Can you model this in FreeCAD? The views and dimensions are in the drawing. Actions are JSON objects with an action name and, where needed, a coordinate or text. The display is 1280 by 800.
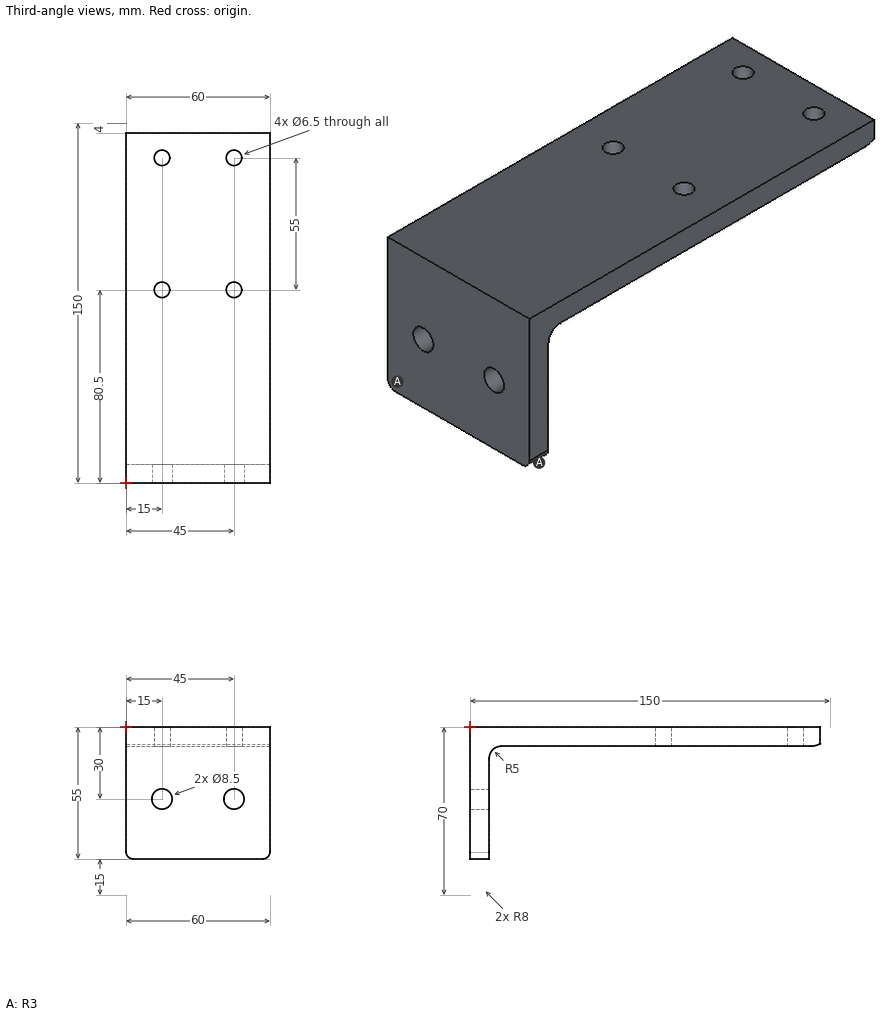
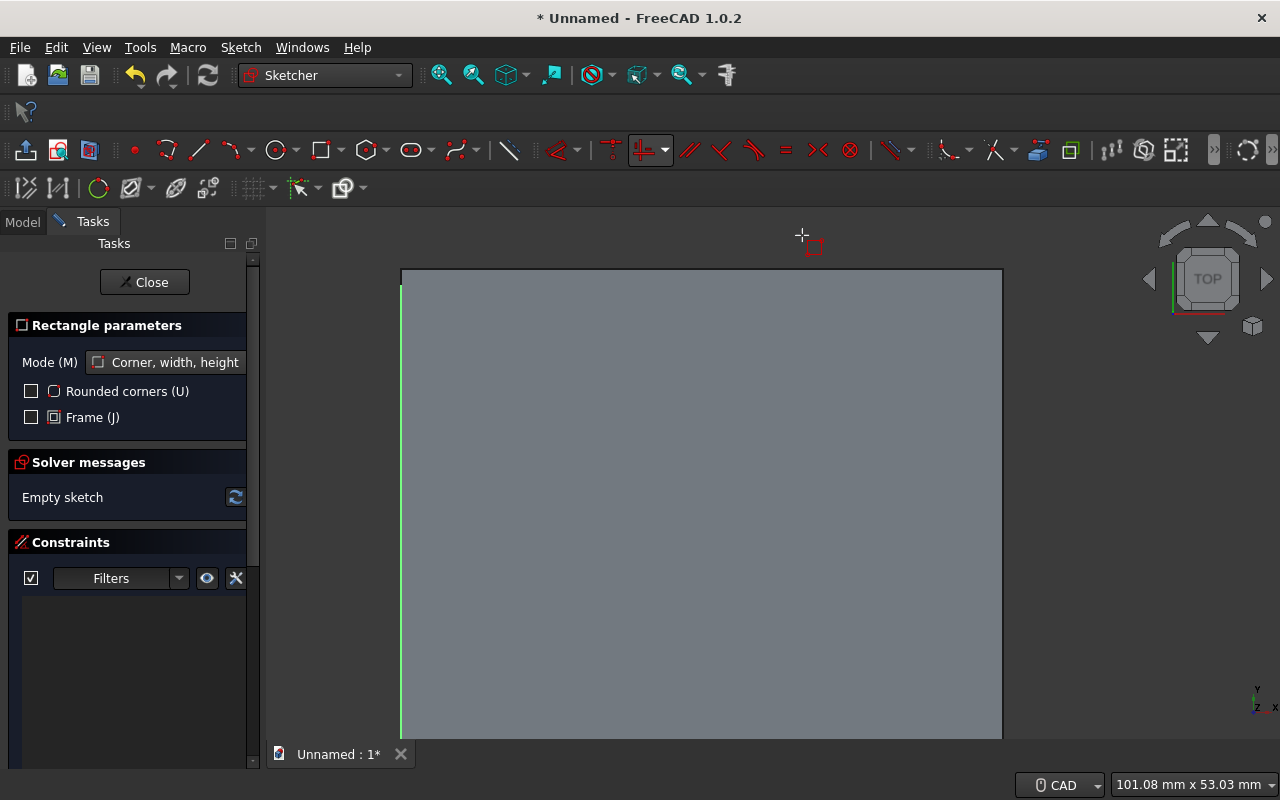
{"action": "left_click", "coordinate": [401, 269]}
{"action": "left_click", "coordinate": [1003, 309]}
{"action": "key", "text": "Escape"}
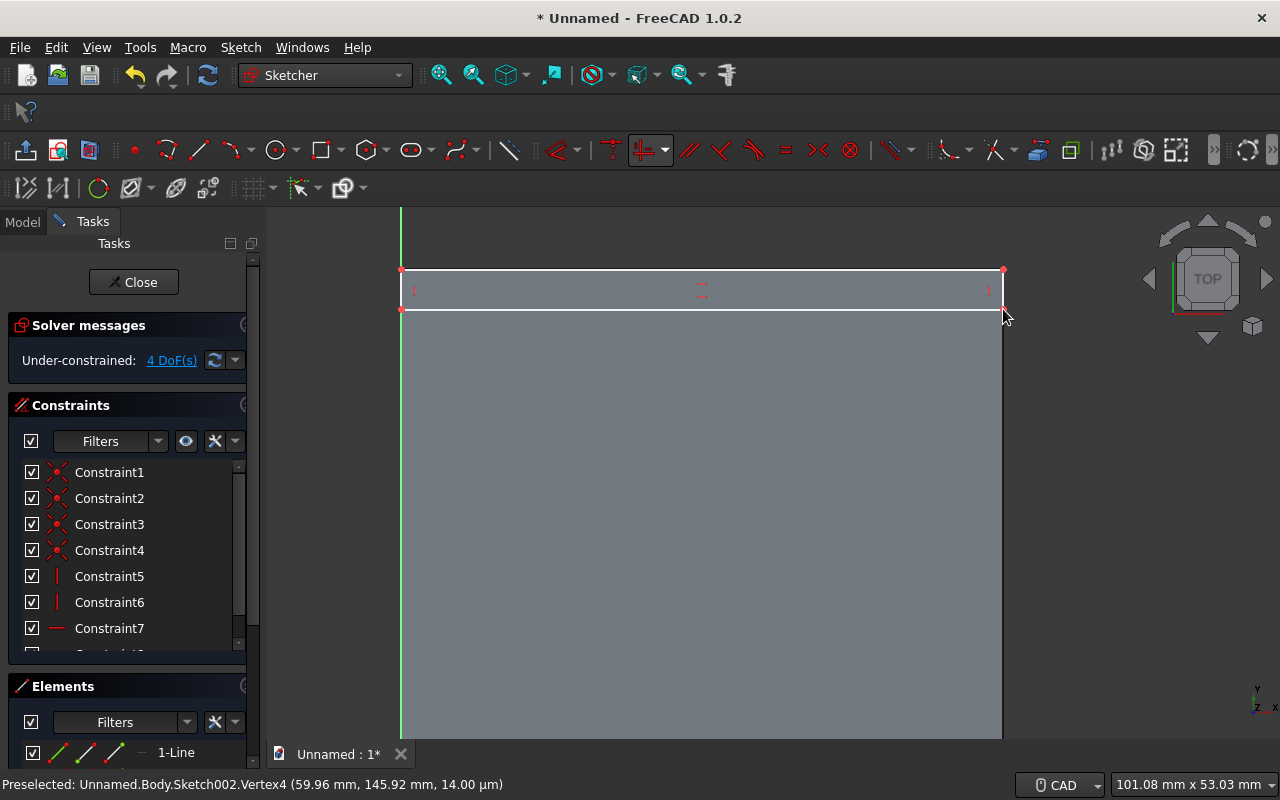
{"action": "left_click", "coordinate": [401, 270]}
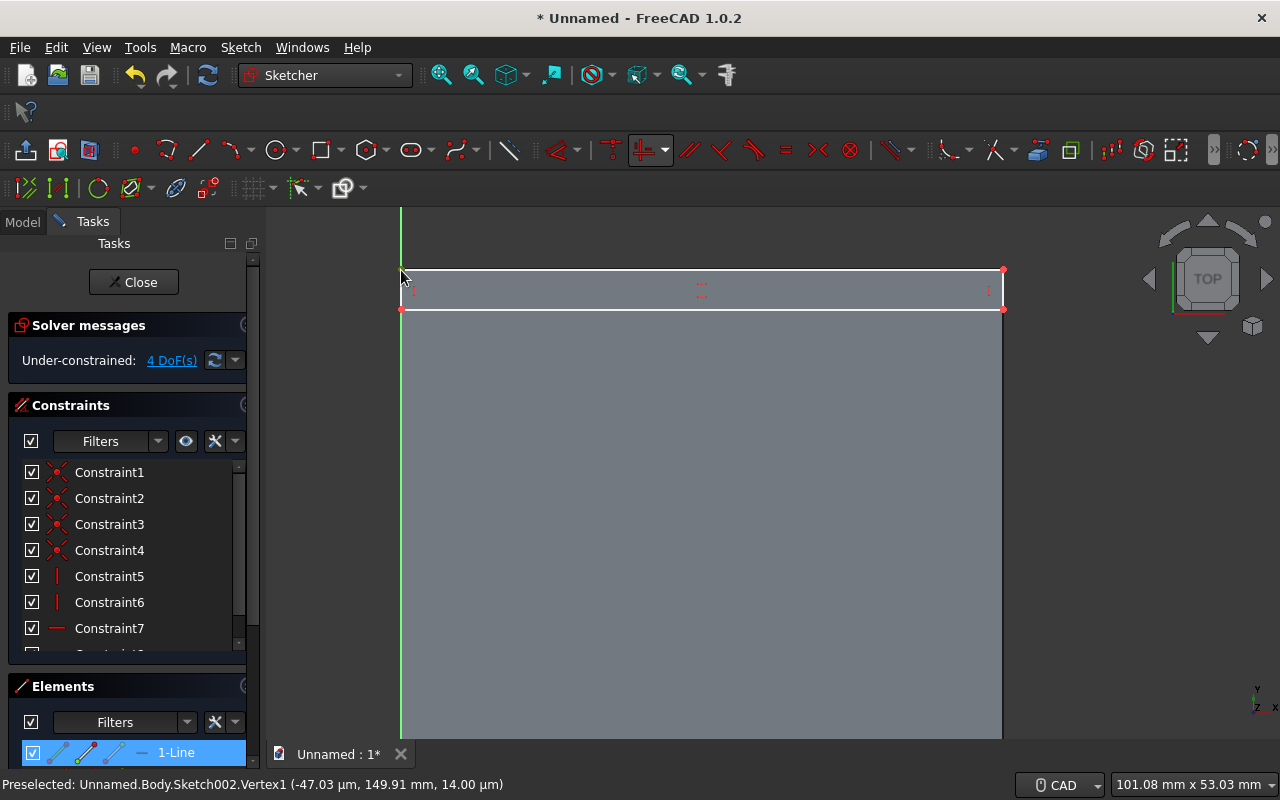
{"action": "left_click", "coordinate": [401, 677]}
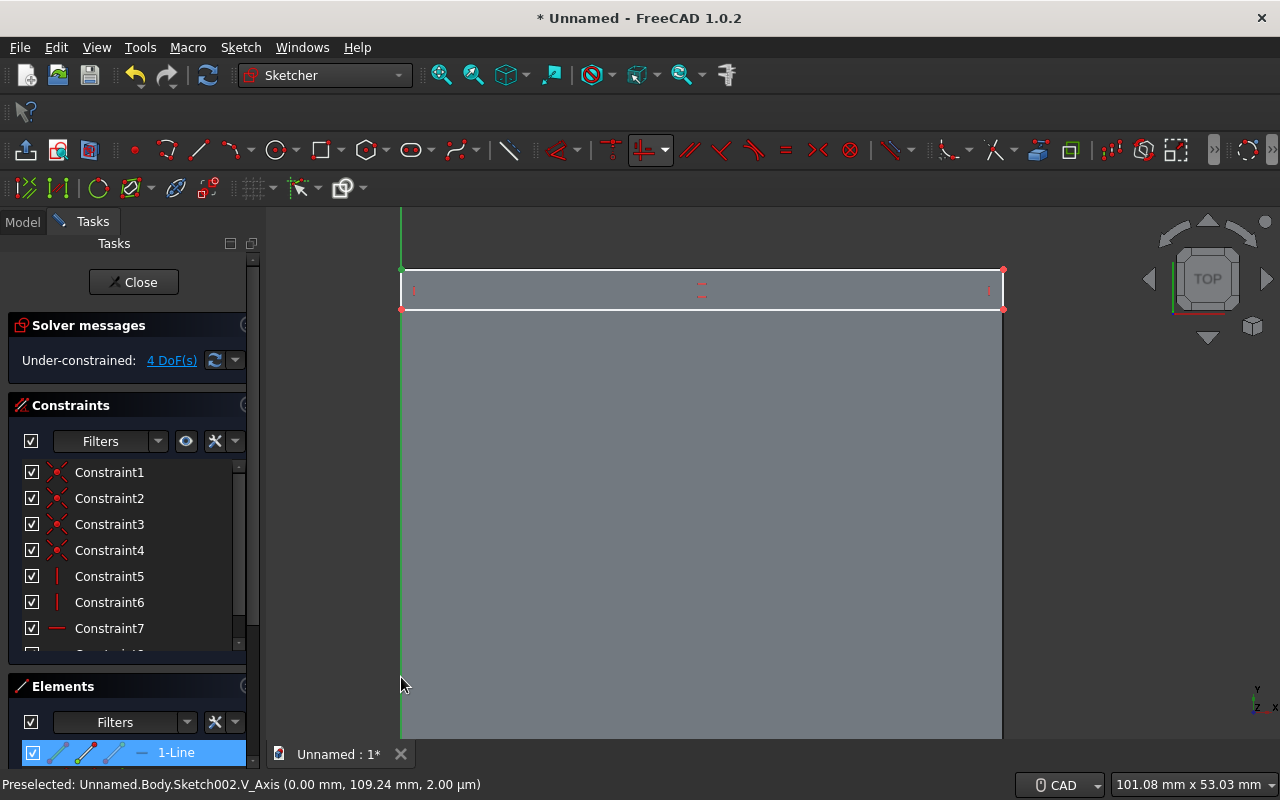
{"action": "key", "text": "c"}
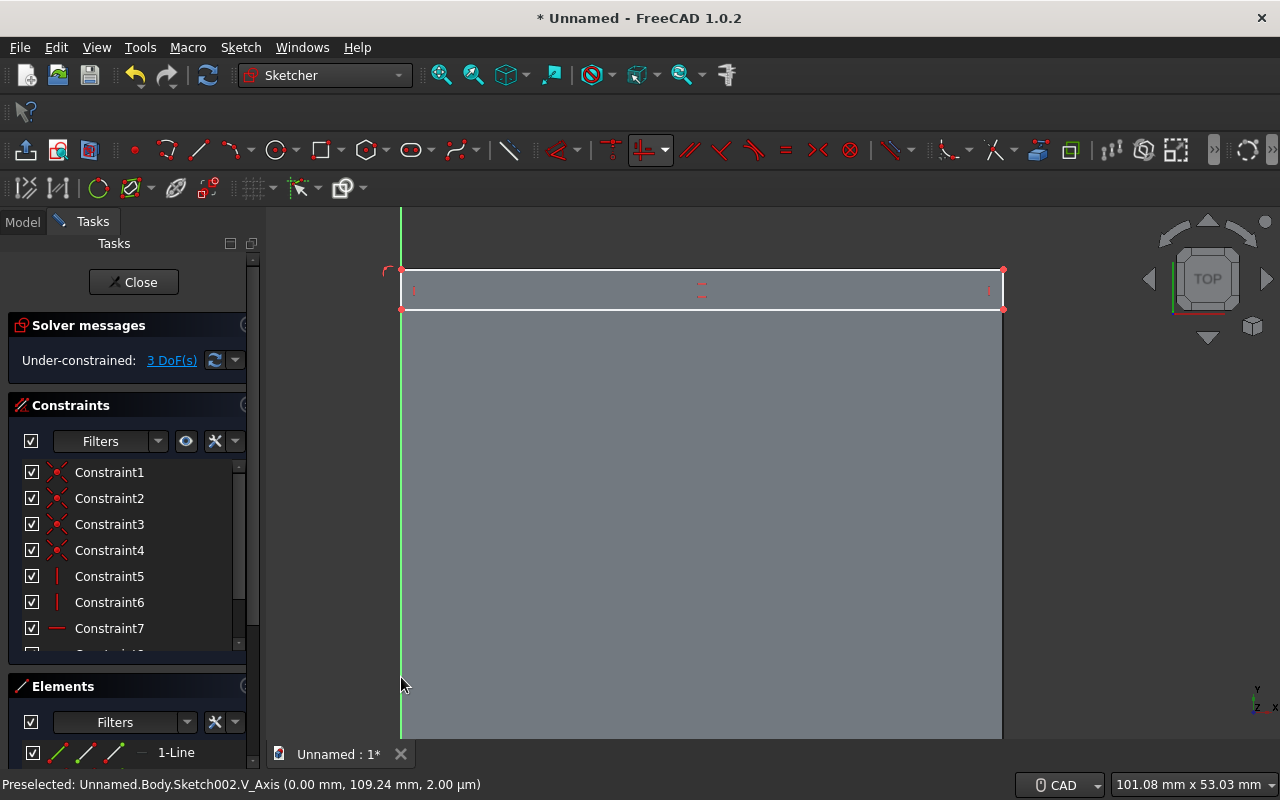
{"action": "key", "text": "d"}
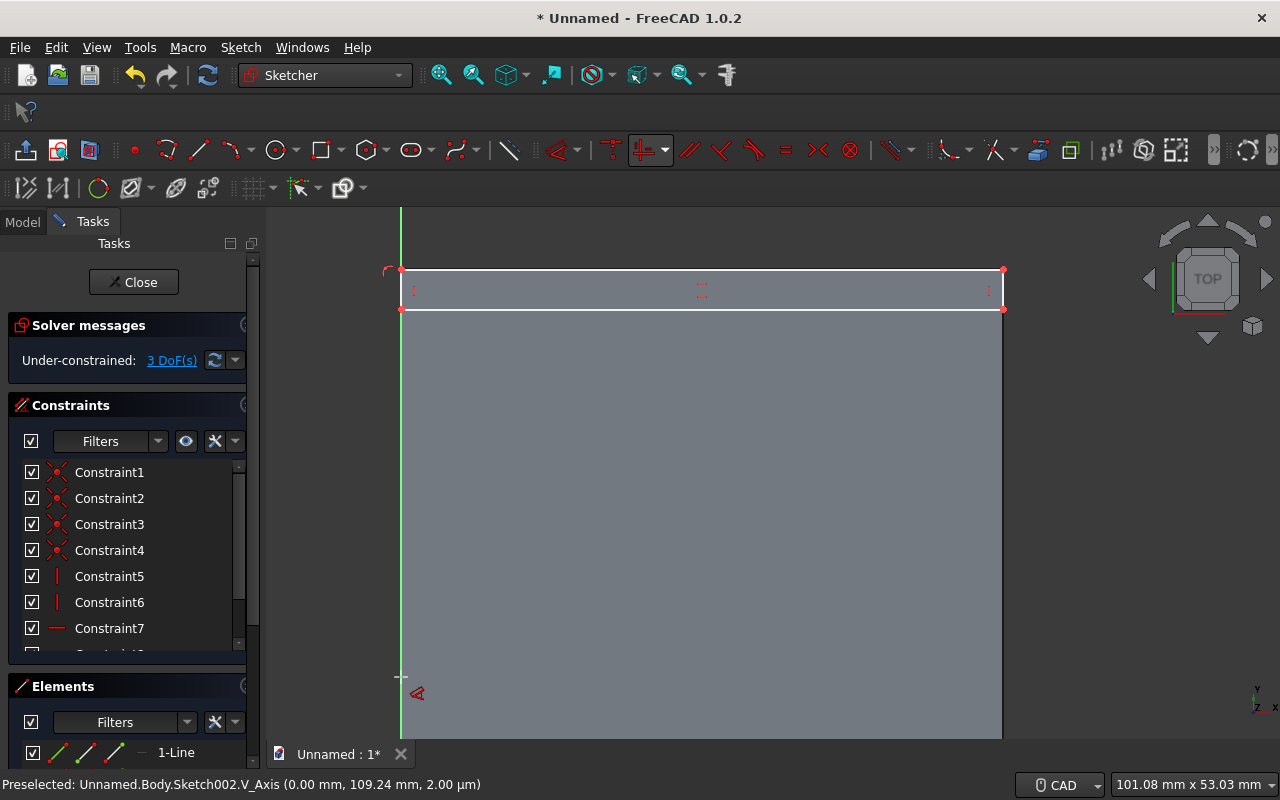
{"action": "left_click", "coordinate": [401, 282]}
{"action": "left_click", "coordinate": [367, 290]}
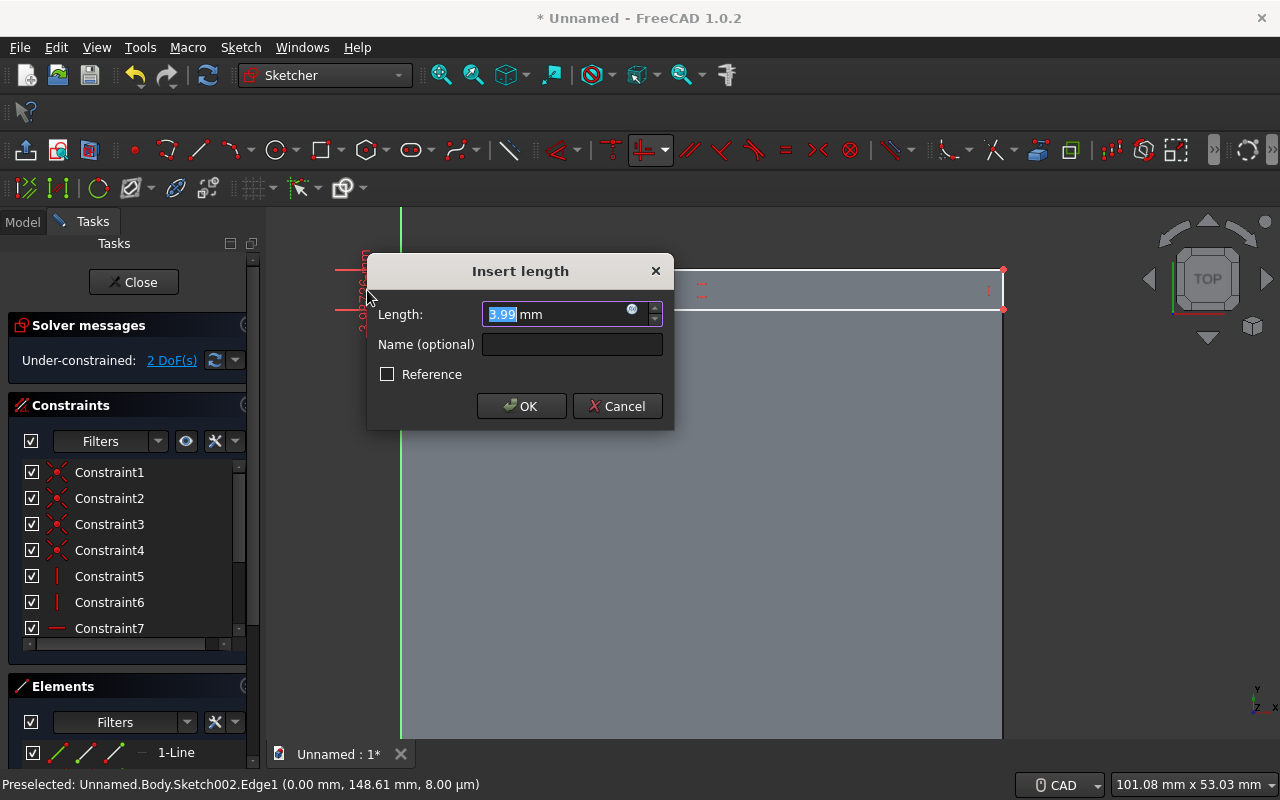
{"action": "type", "text": "4"}
{"action": "key", "text": "Return"}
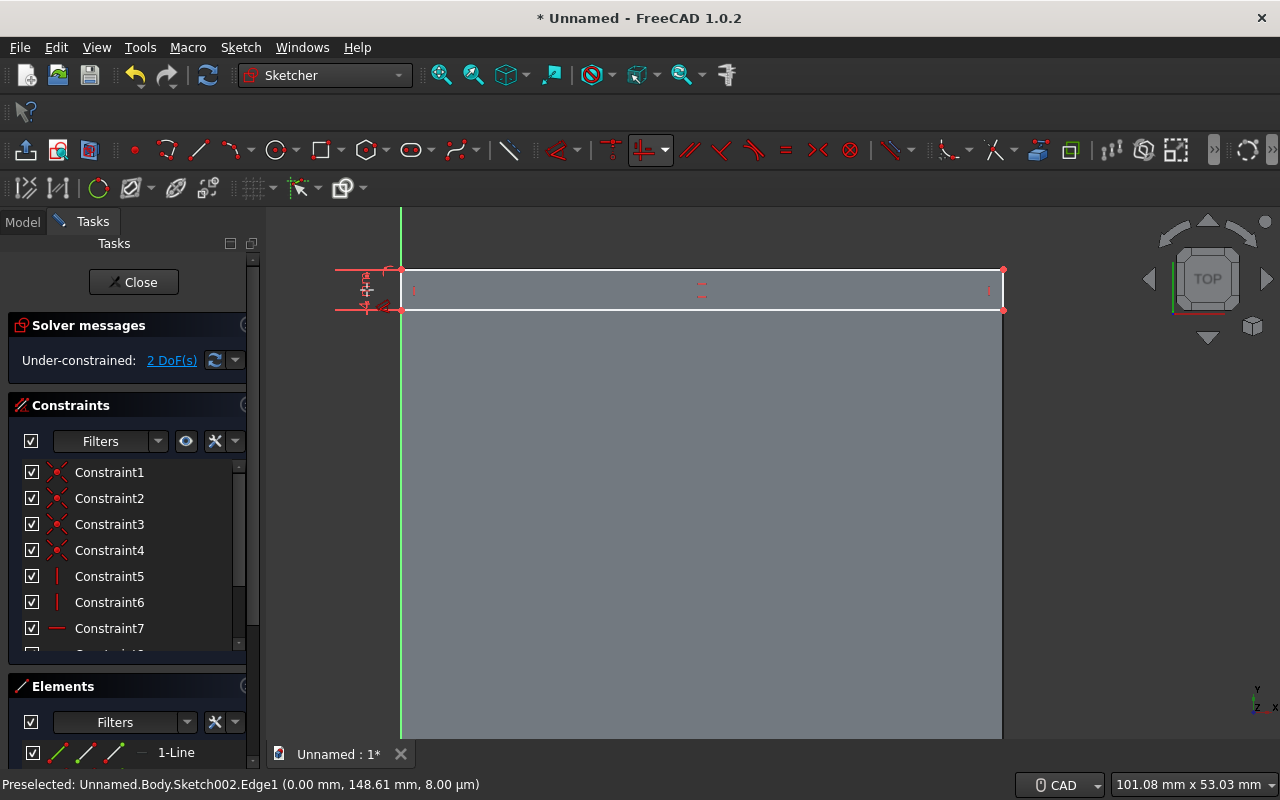
{"action": "left_click", "coordinate": [582, 310]}
{"action": "left_click", "coordinate": [702, 344]}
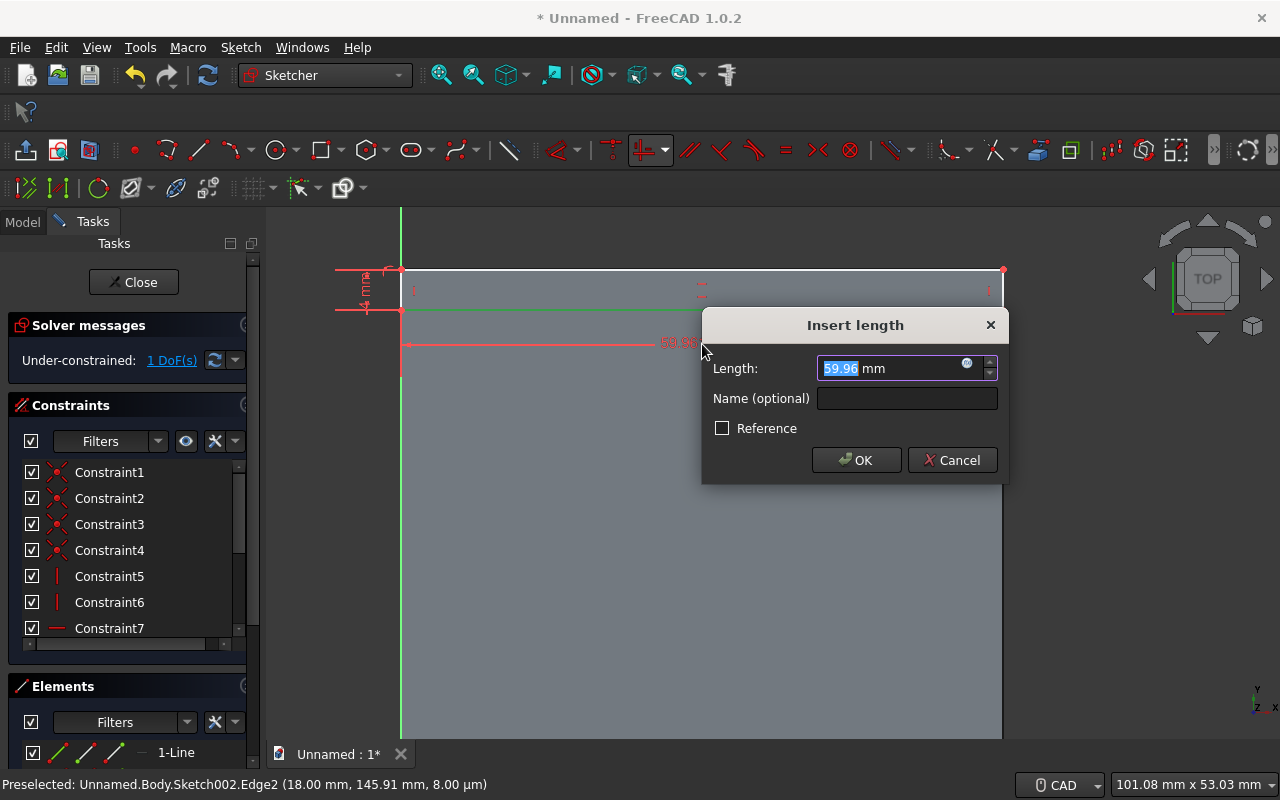
{"action": "type", "text": "60"}
{"action": "key", "text": "Return"}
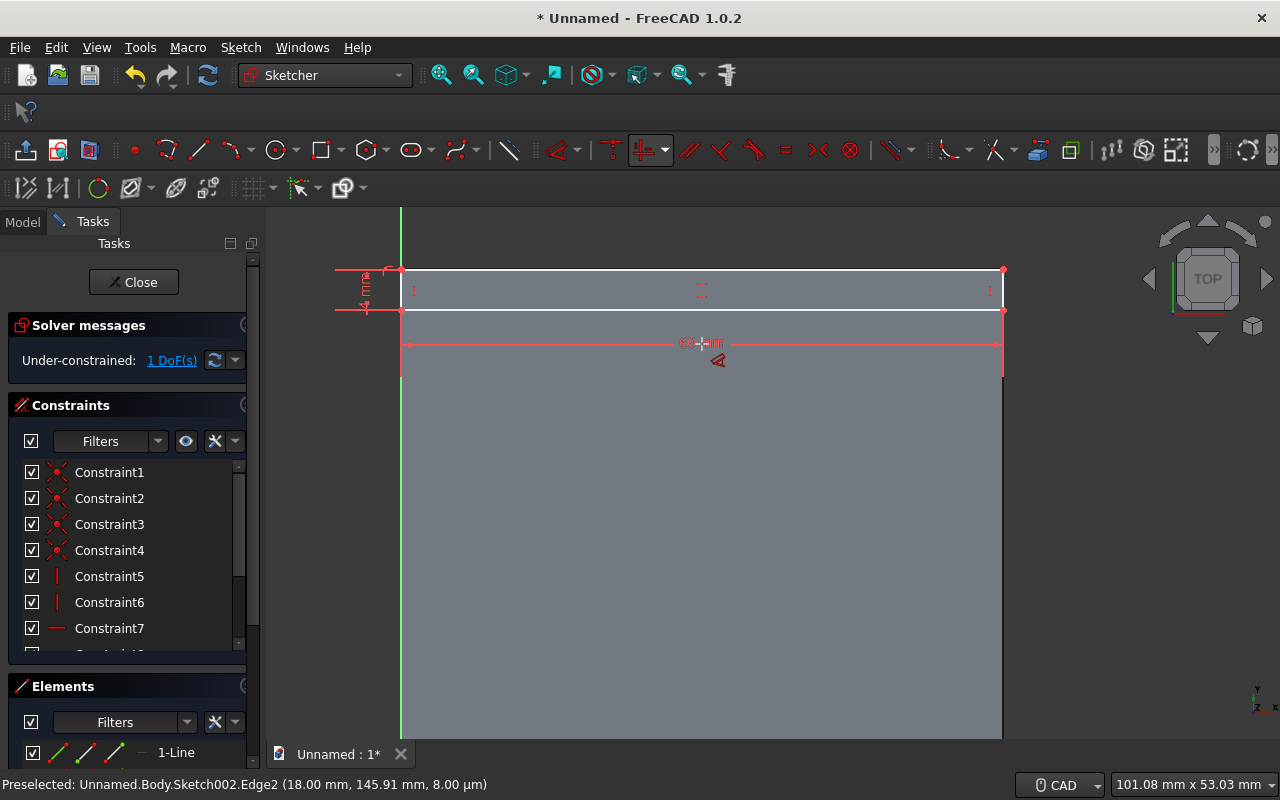
{"action": "left_click", "coordinate": [401, 270]}
{"action": "left_click", "coordinate": [367, 491]}